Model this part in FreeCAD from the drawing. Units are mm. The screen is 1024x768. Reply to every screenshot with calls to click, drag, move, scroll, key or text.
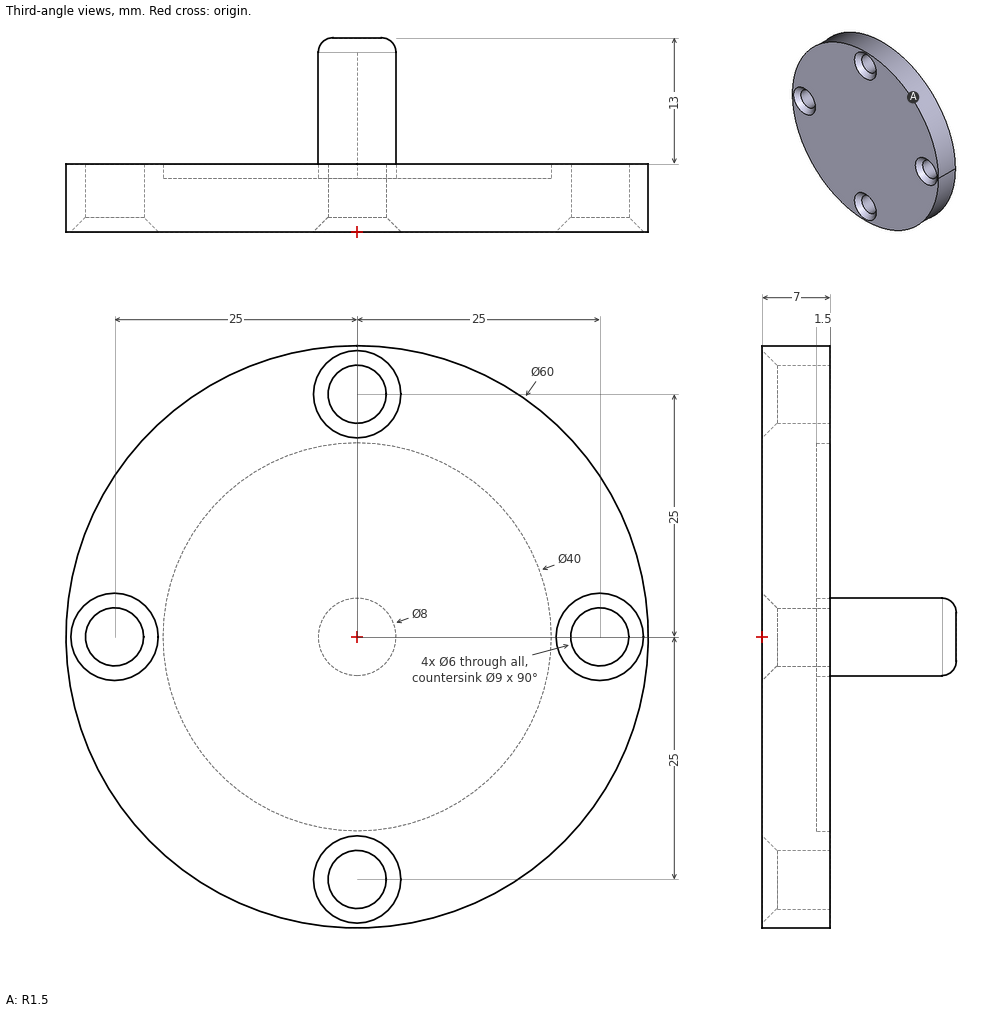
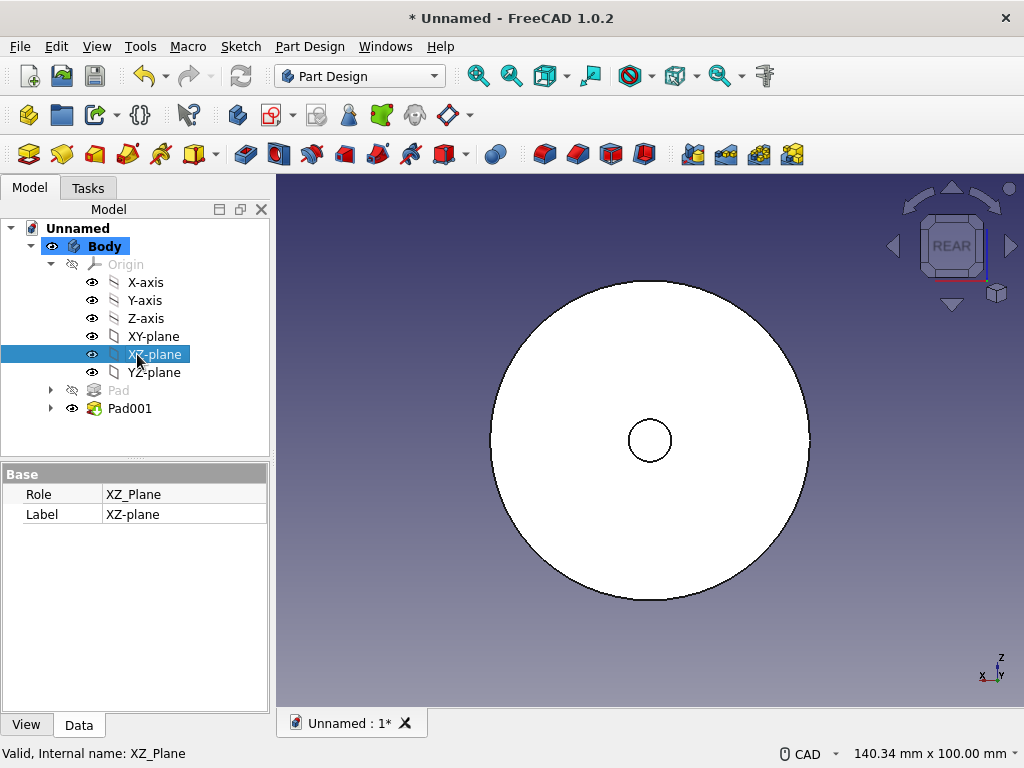
click(448, 116)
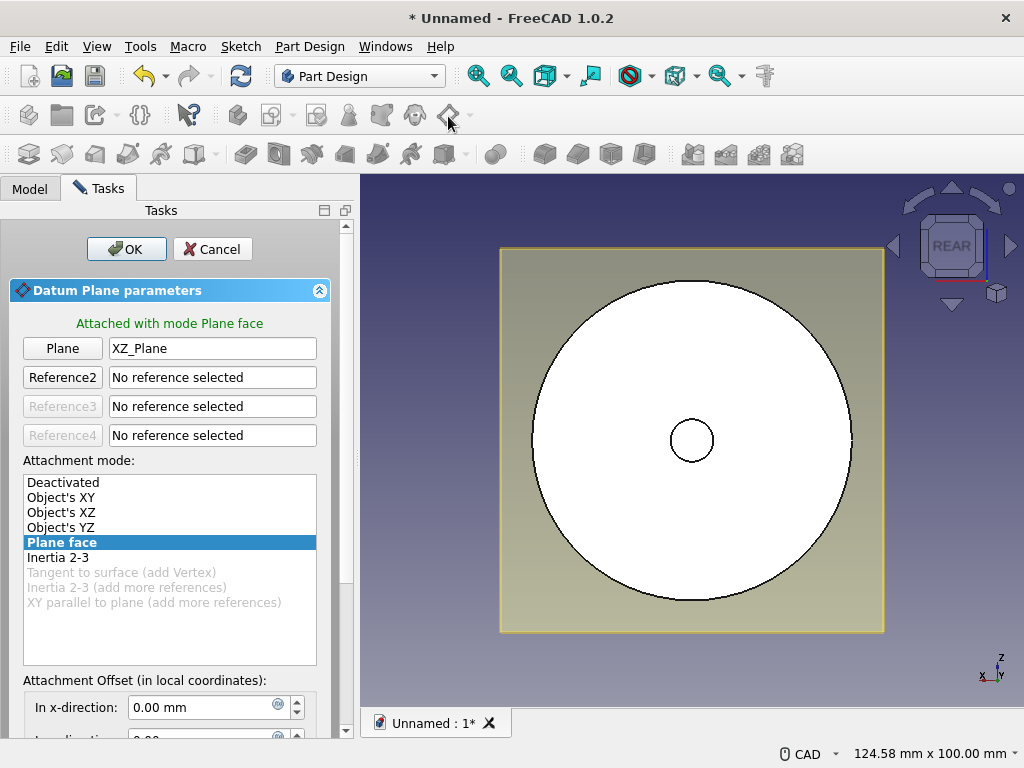
scroll(346, 479, down, 2)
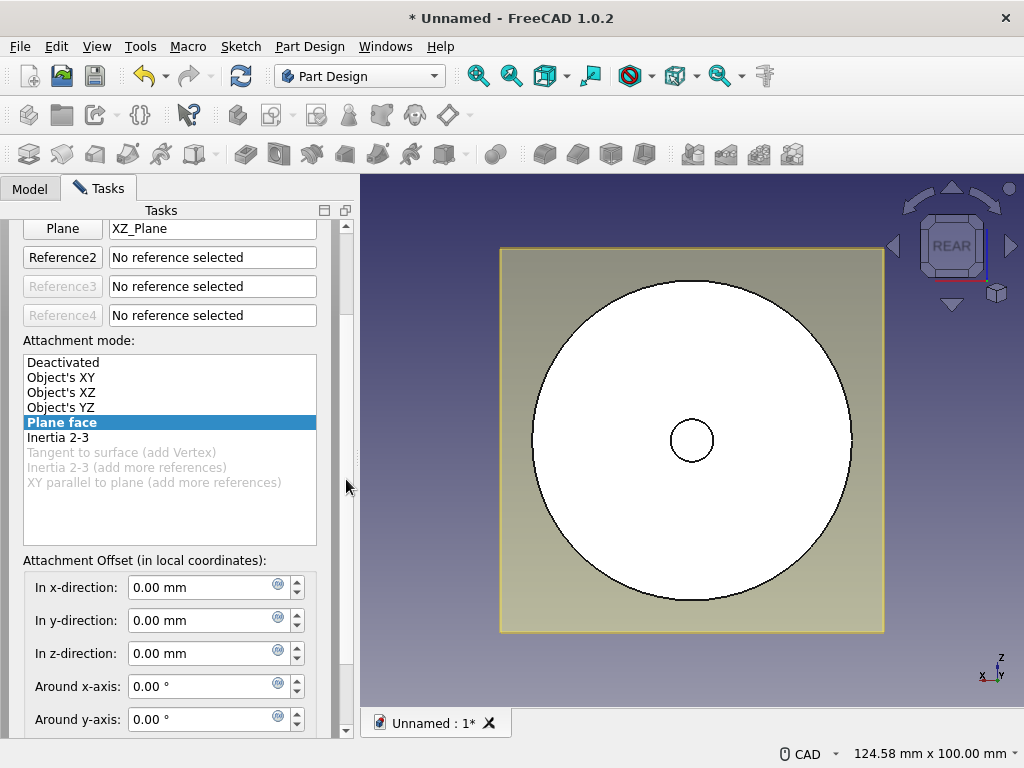
triple_click(210, 654)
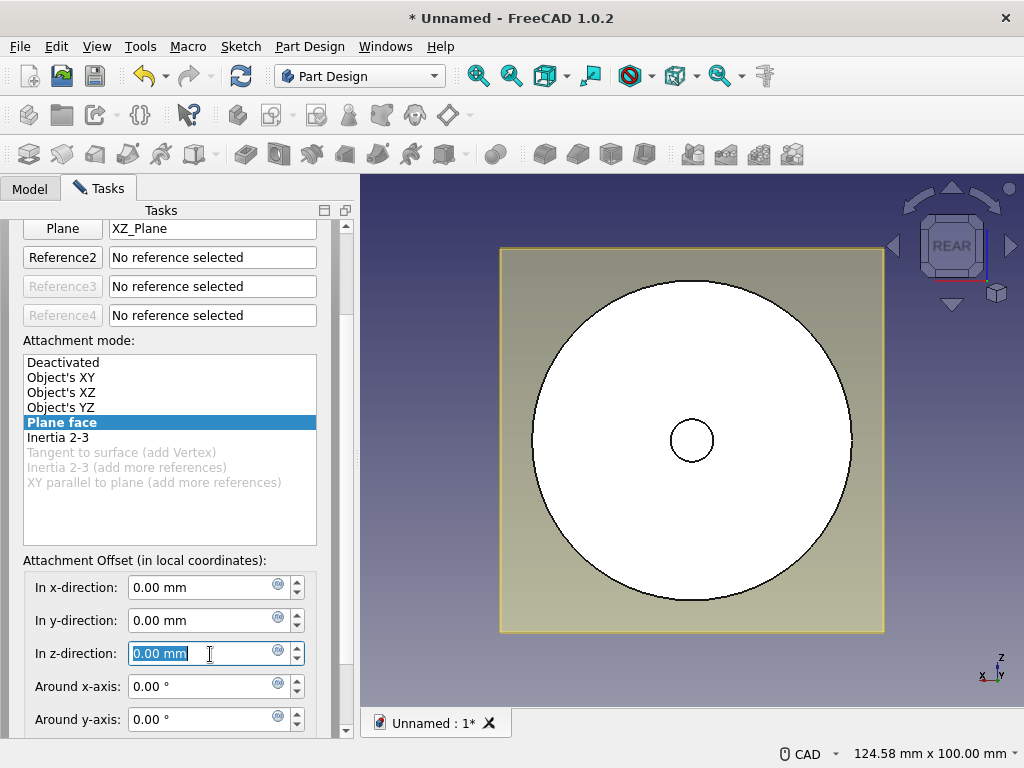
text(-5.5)
key(Tab)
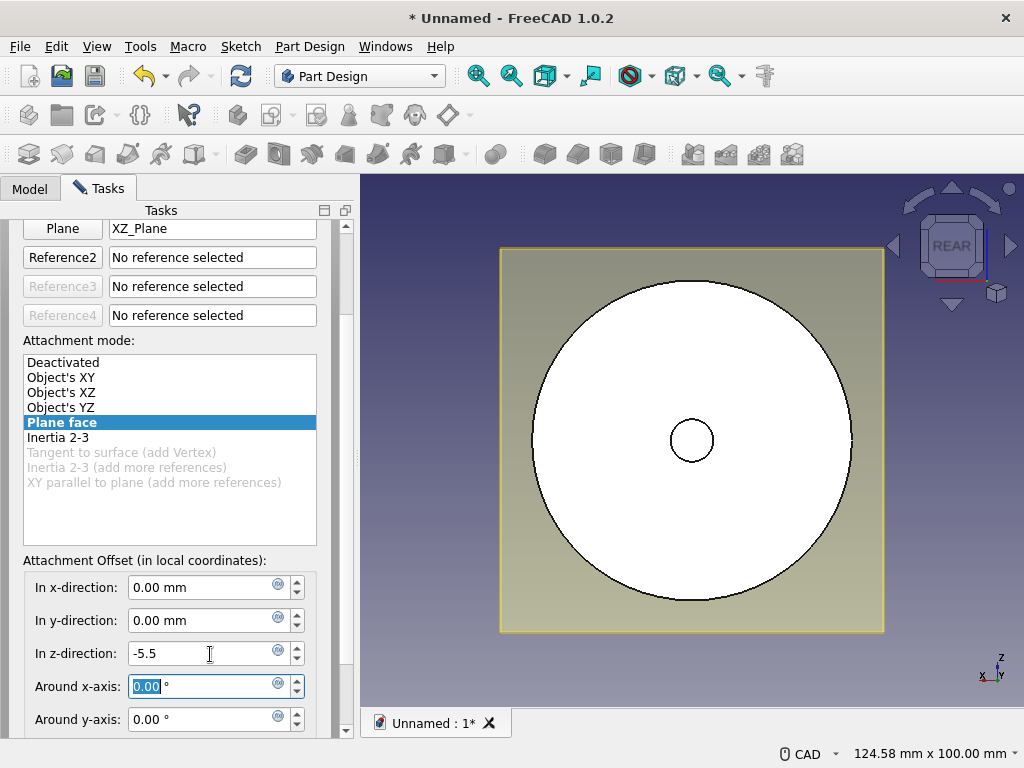
scroll(346, 479, up, 3)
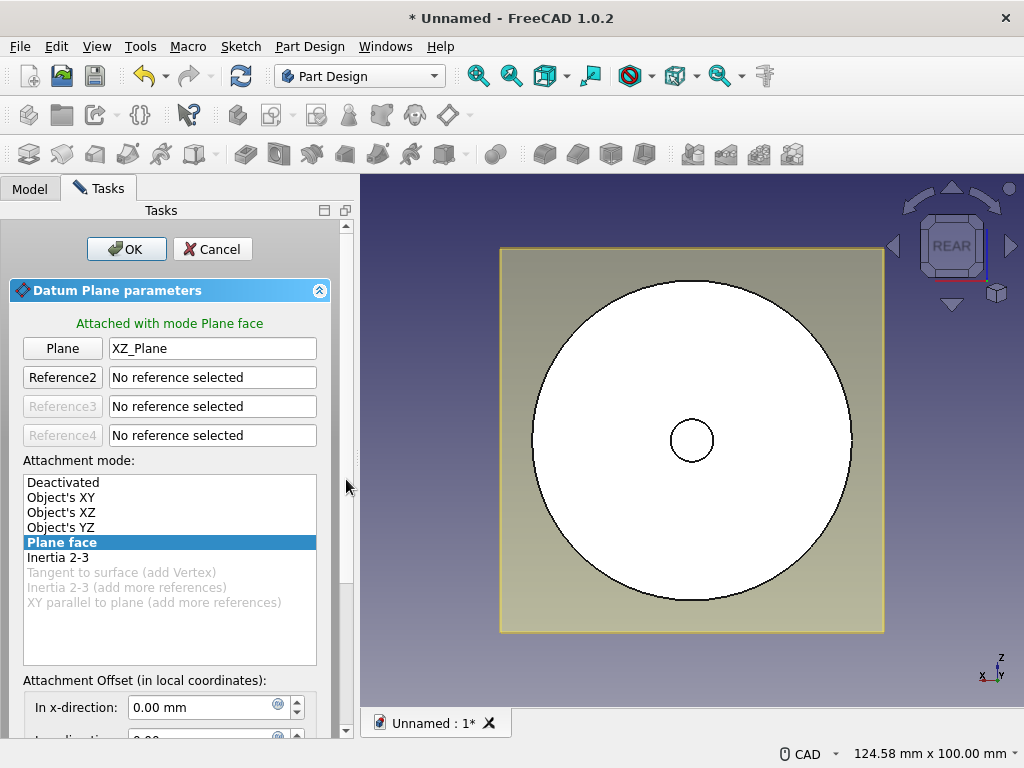
click(127, 249)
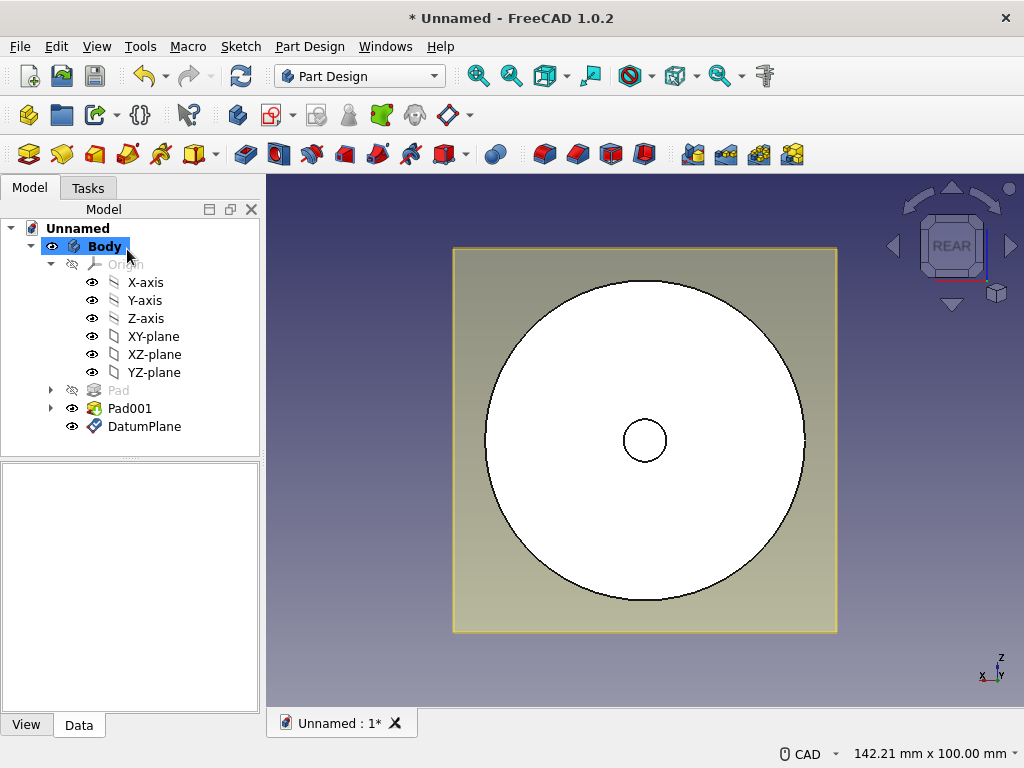
click(117, 426)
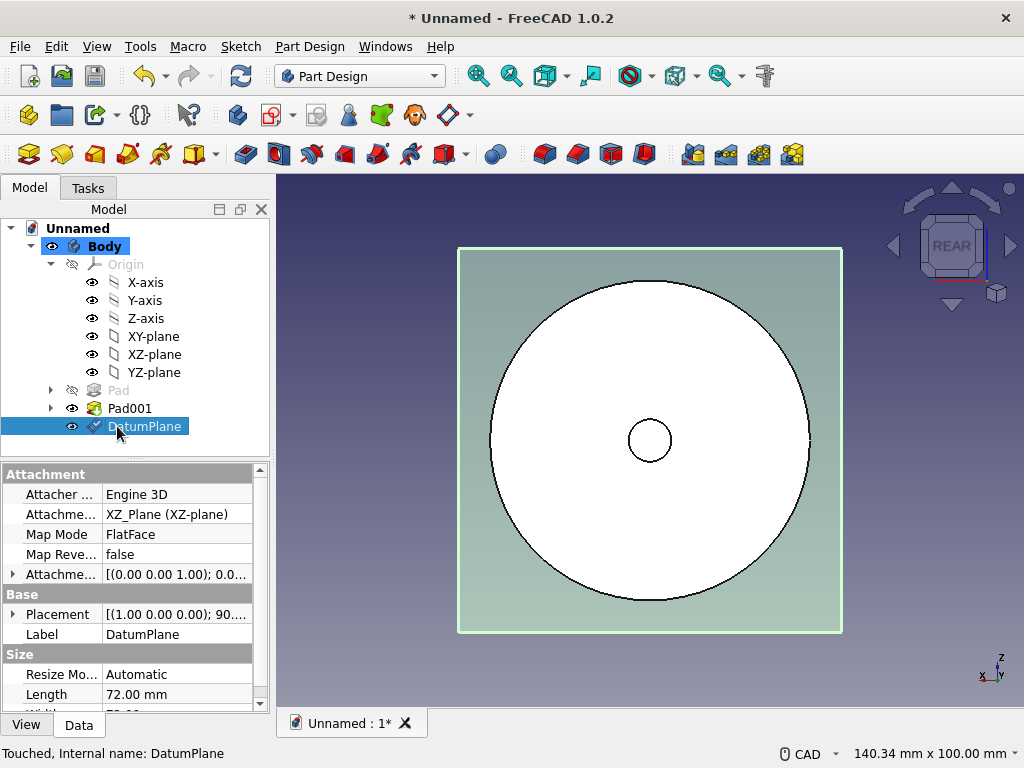
click(270, 116)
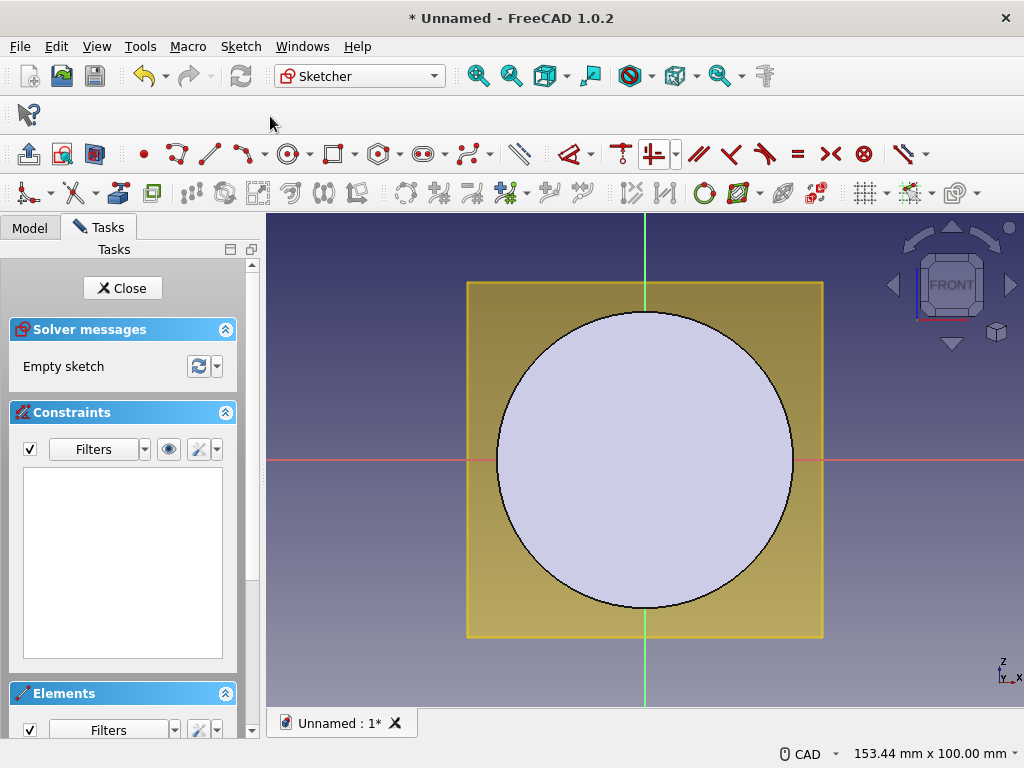
click(95, 154)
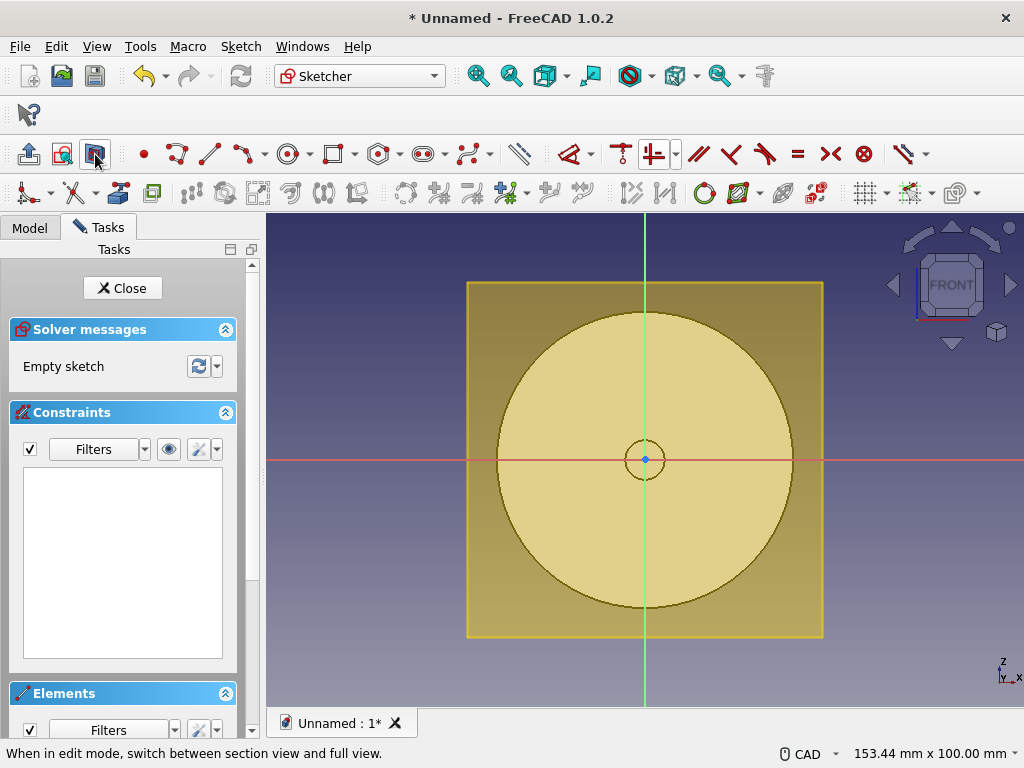
scroll(784, 460, up, 2)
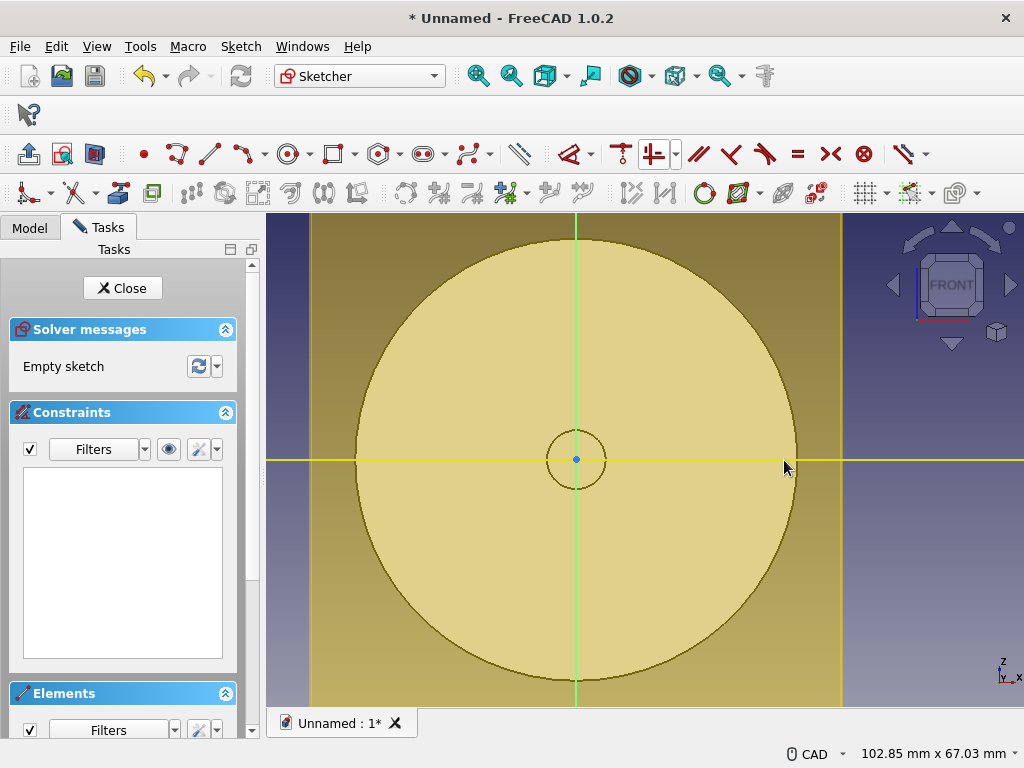
click(288, 154)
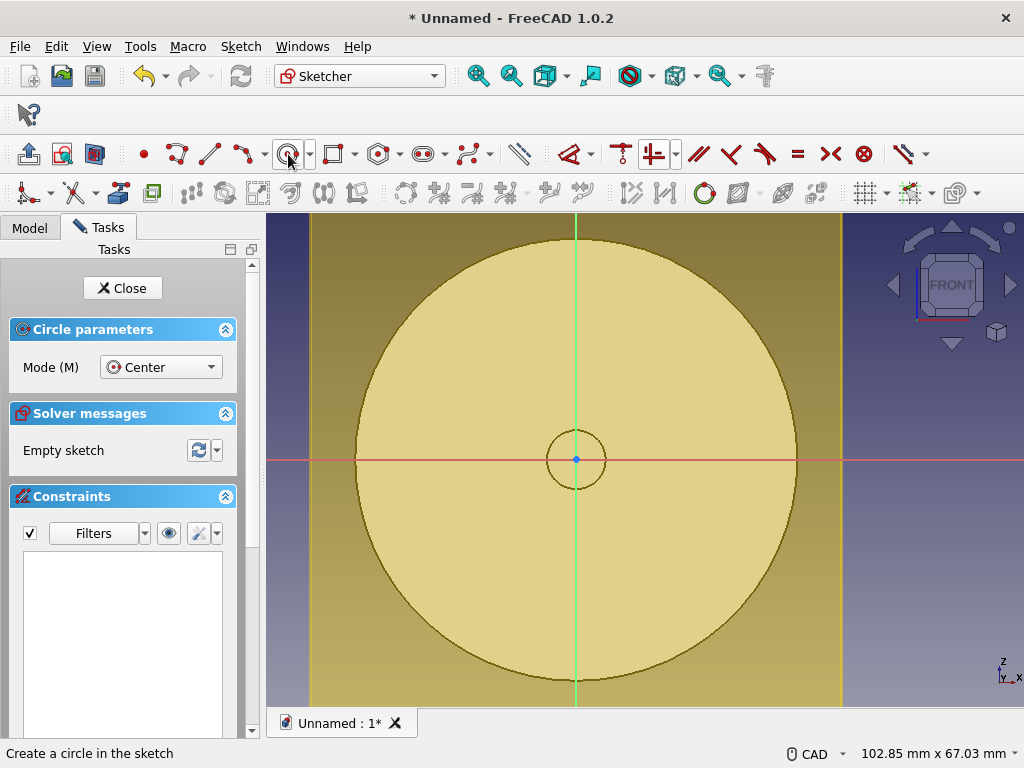
click(576, 460)
move(681, 356)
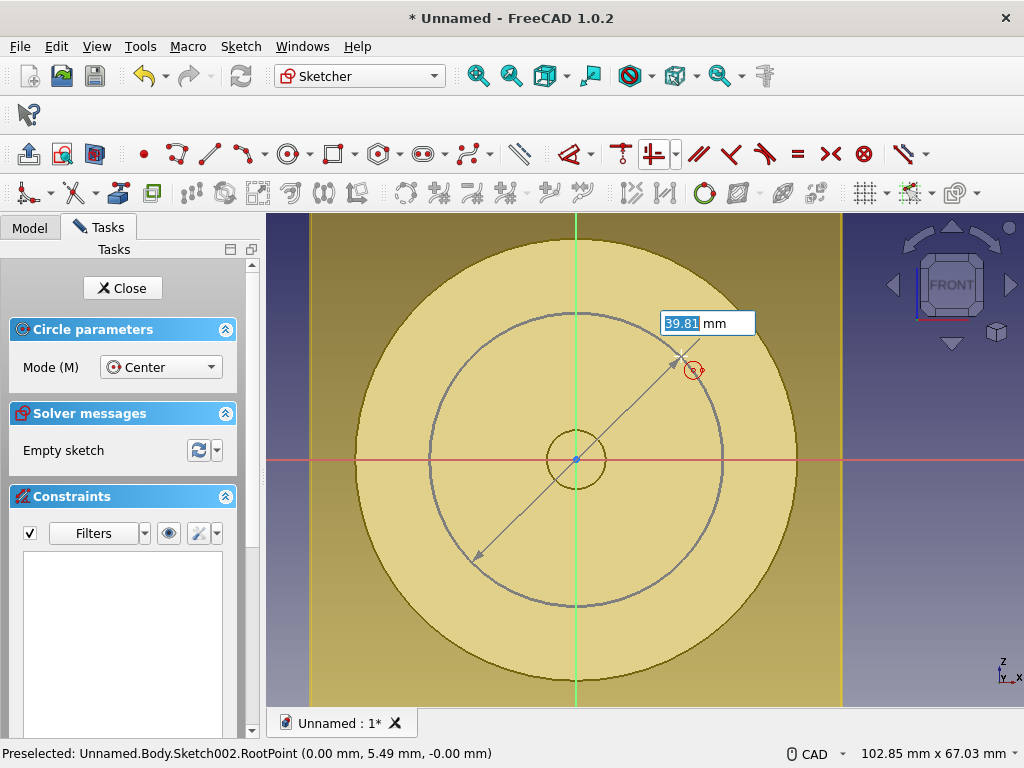
text(40)
key(Return)